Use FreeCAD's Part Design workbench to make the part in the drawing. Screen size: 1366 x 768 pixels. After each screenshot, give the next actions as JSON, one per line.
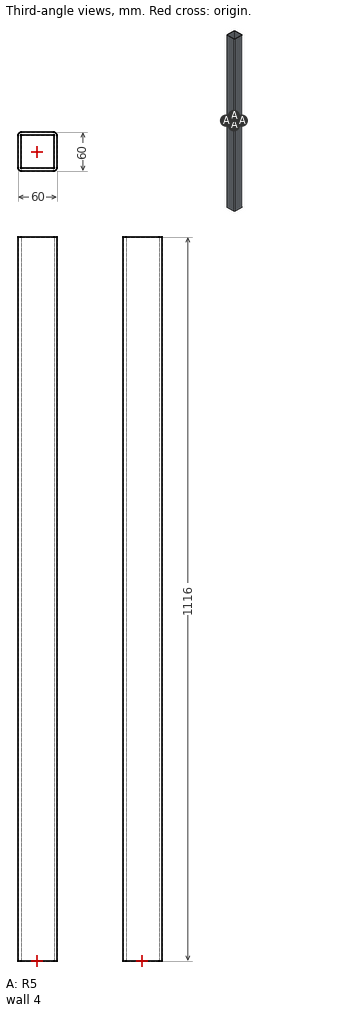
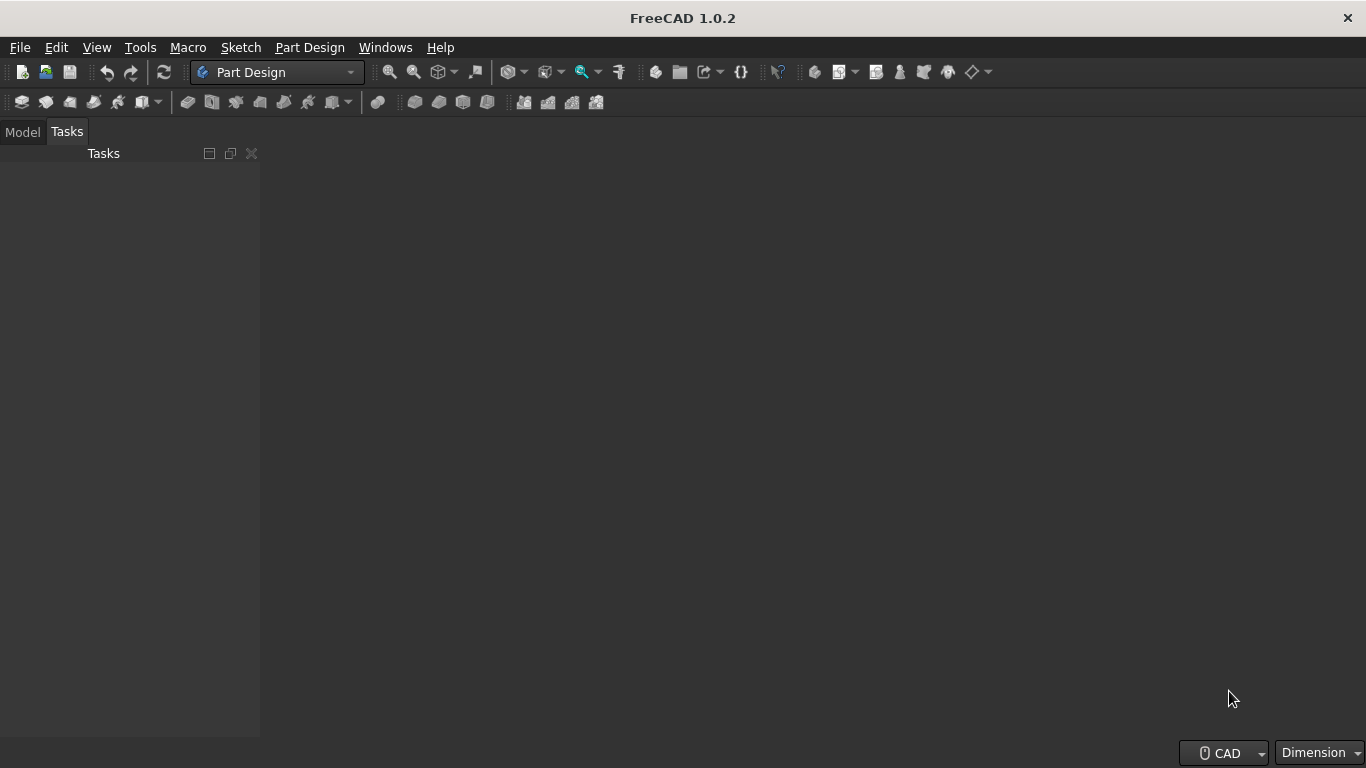
{"action": "left_click", "coordinate": [22, 72]}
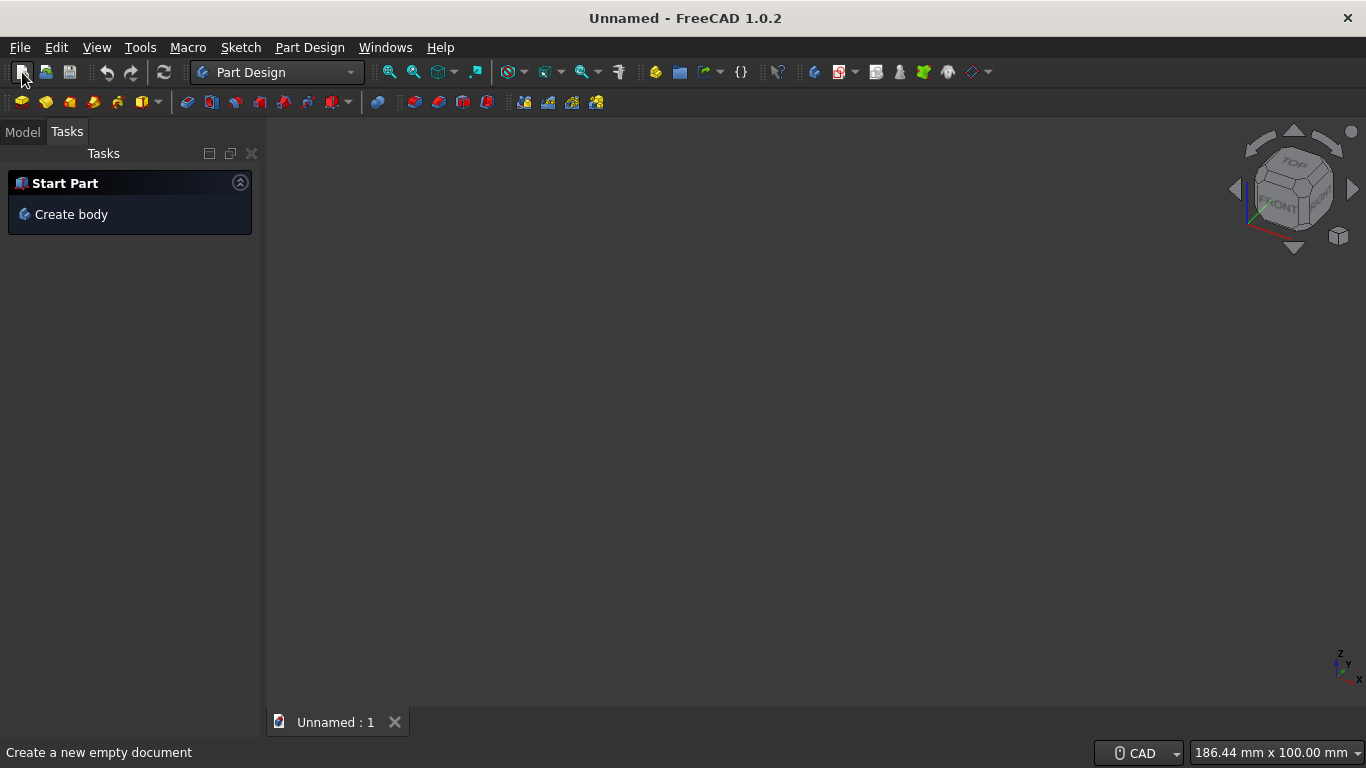
{"action": "left_click", "coordinate": [840, 72]}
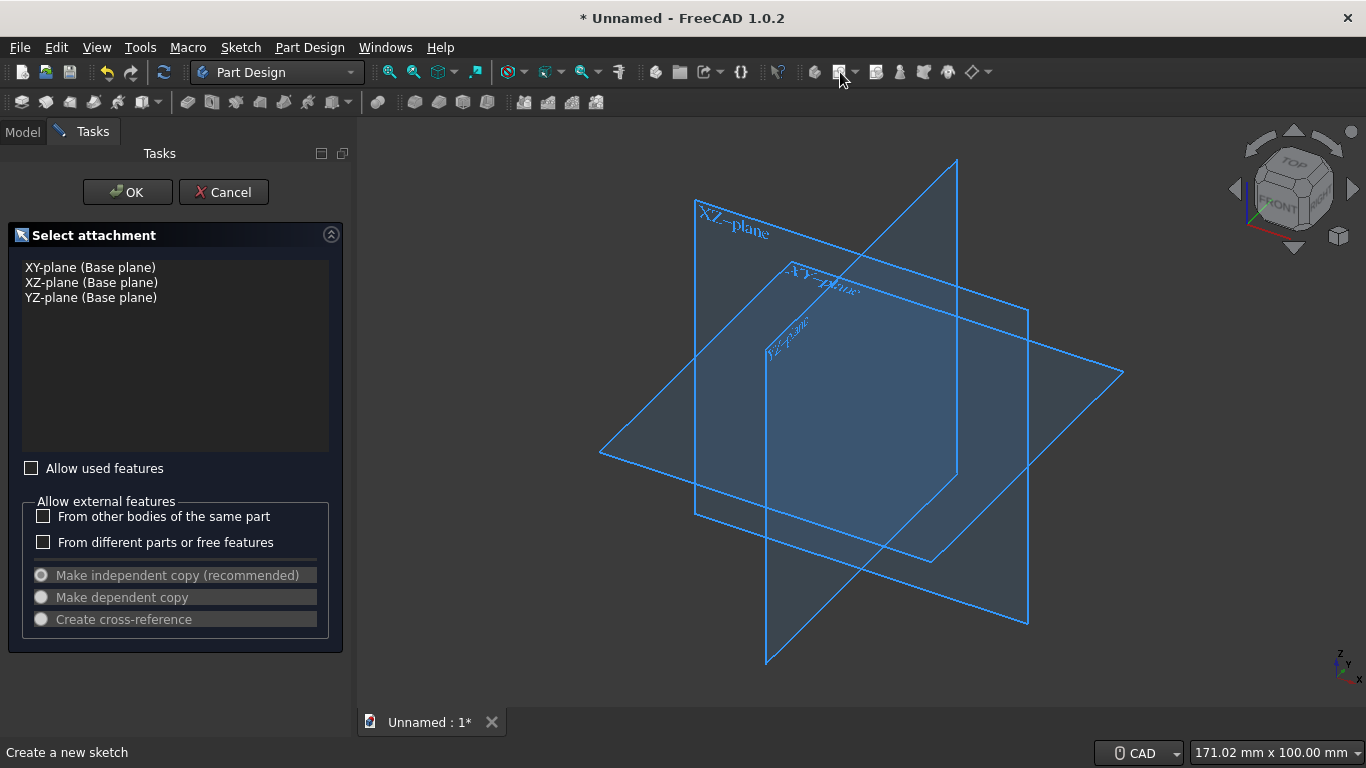
{"action": "left_click", "coordinate": [82, 268]}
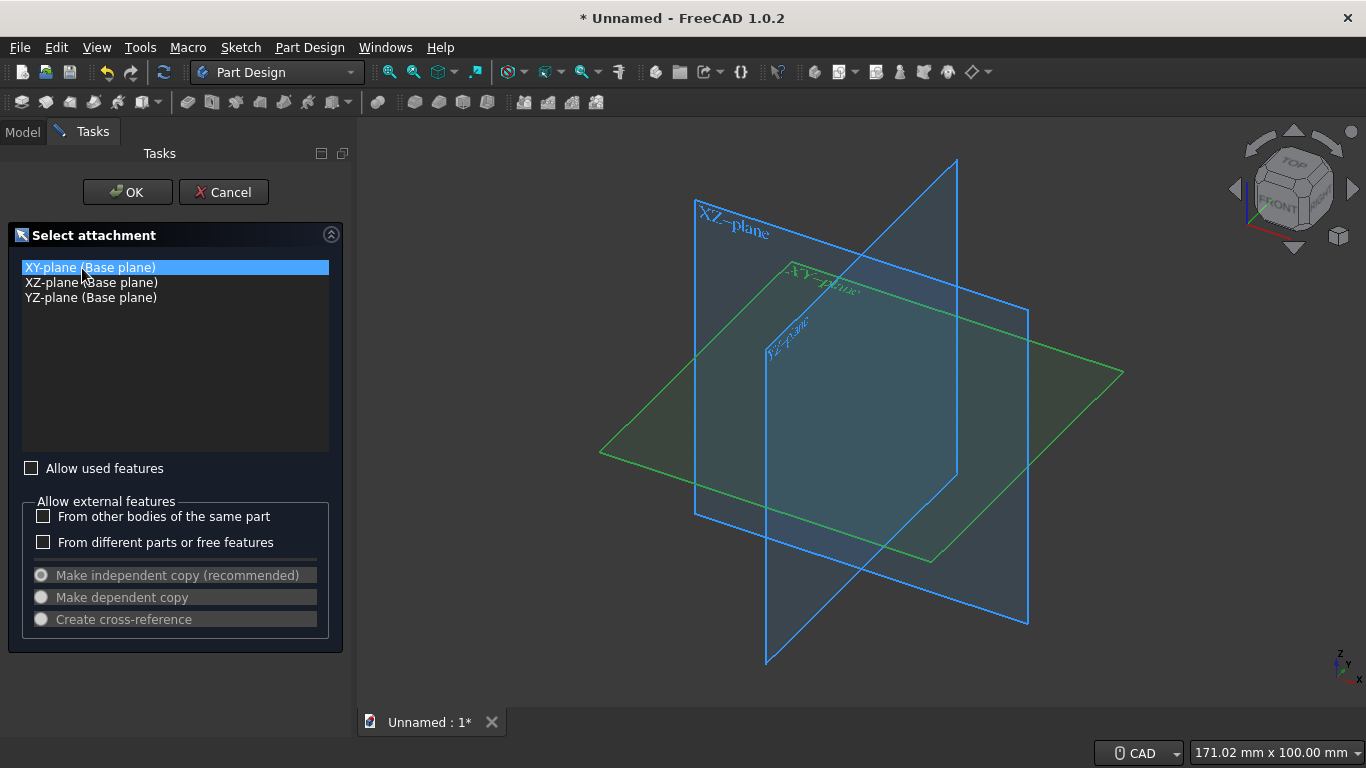
{"action": "left_click", "coordinate": [128, 192]}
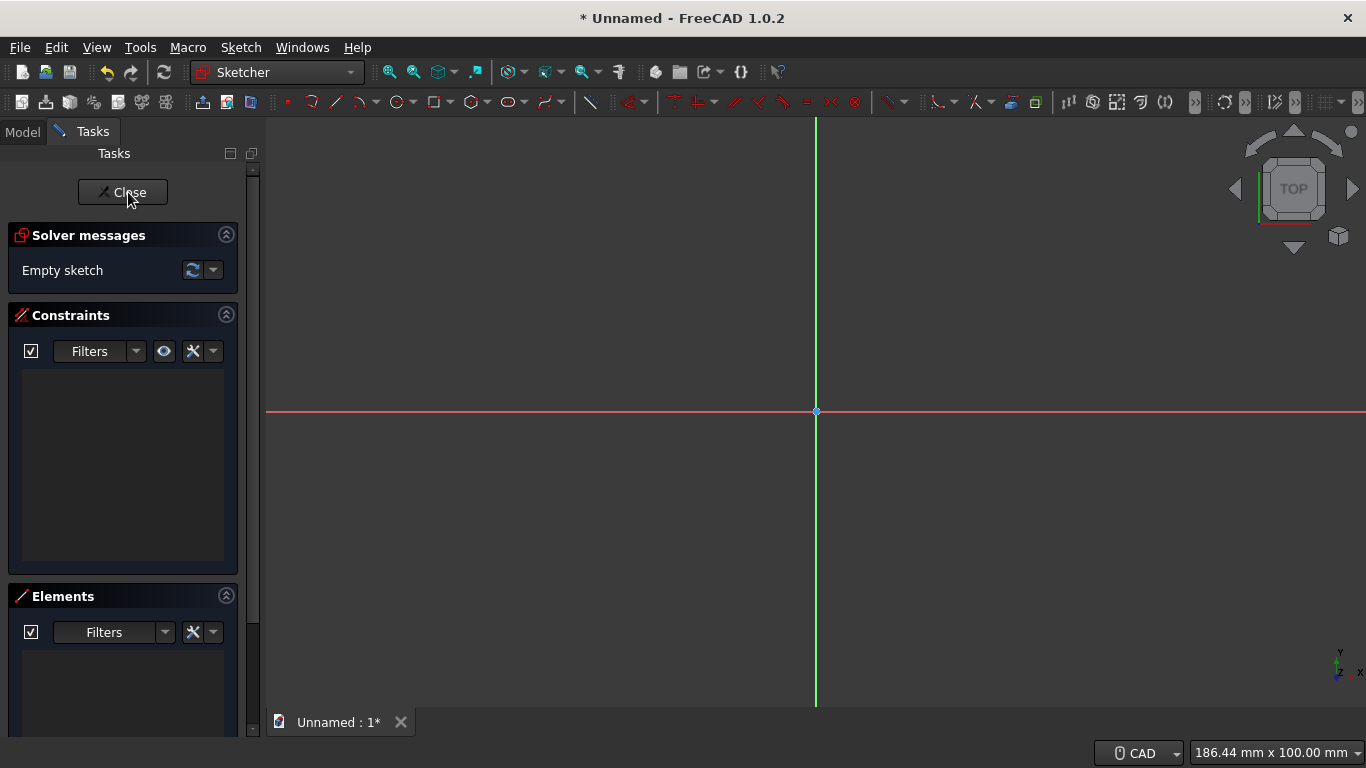
{"action": "left_click", "coordinate": [452, 102]}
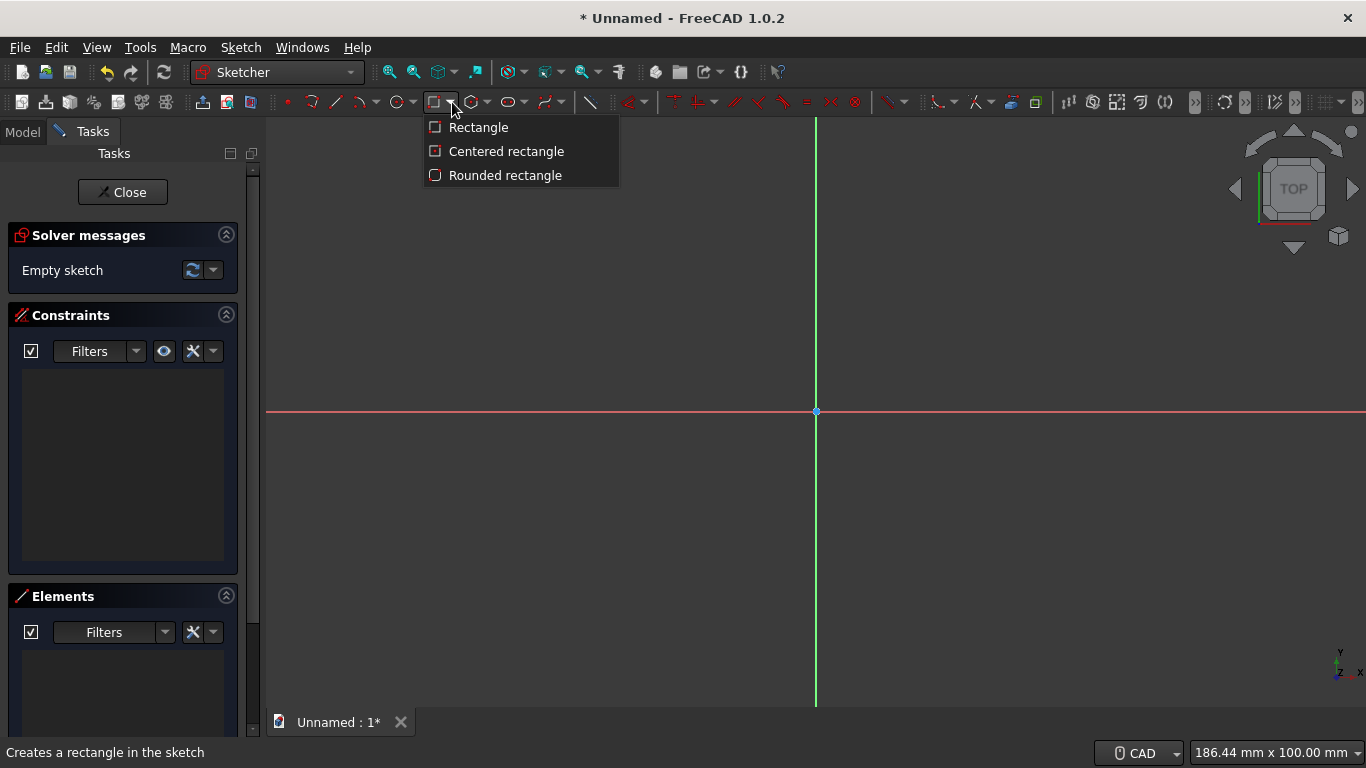
{"action": "left_click", "coordinate": [522, 151]}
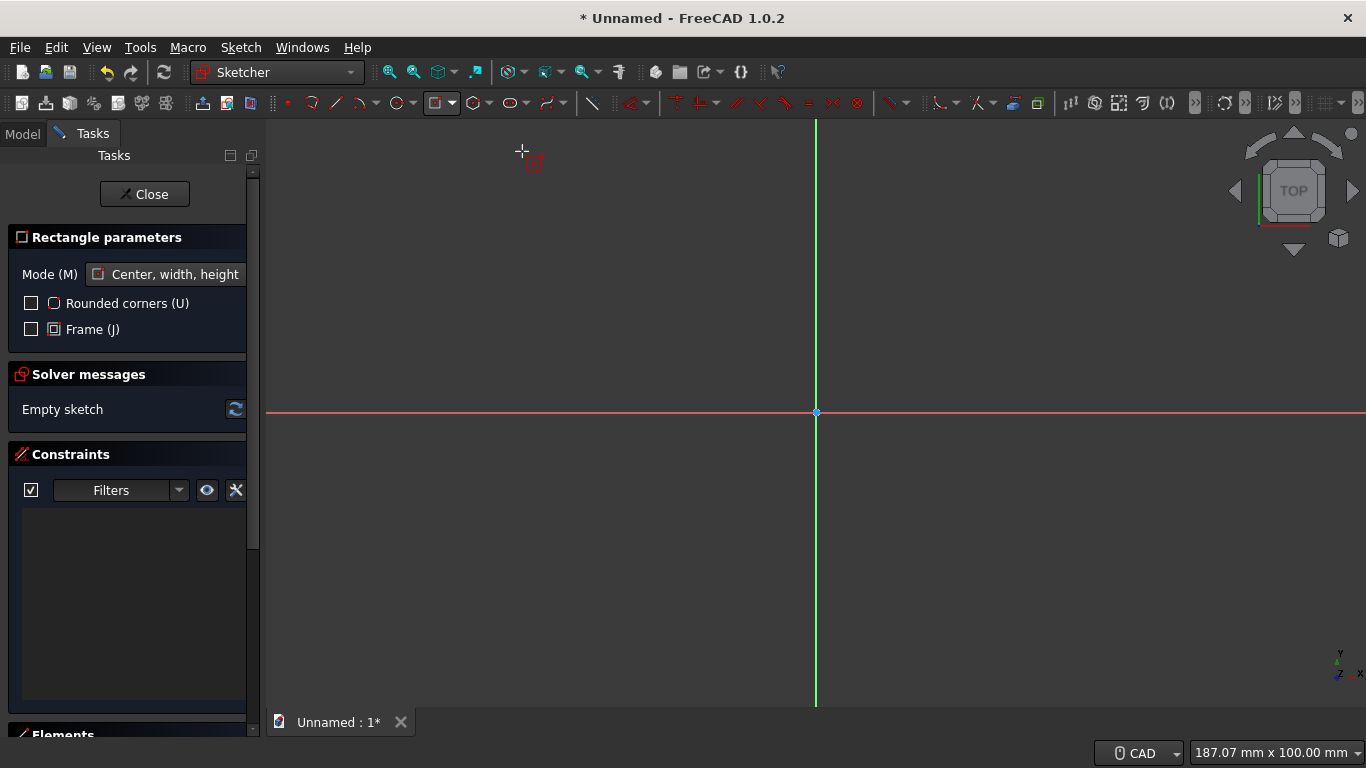
{"action": "left_click", "coordinate": [816, 413]}
{"action": "left_click", "coordinate": [992, 237]}
{"action": "key", "text": "Escape"}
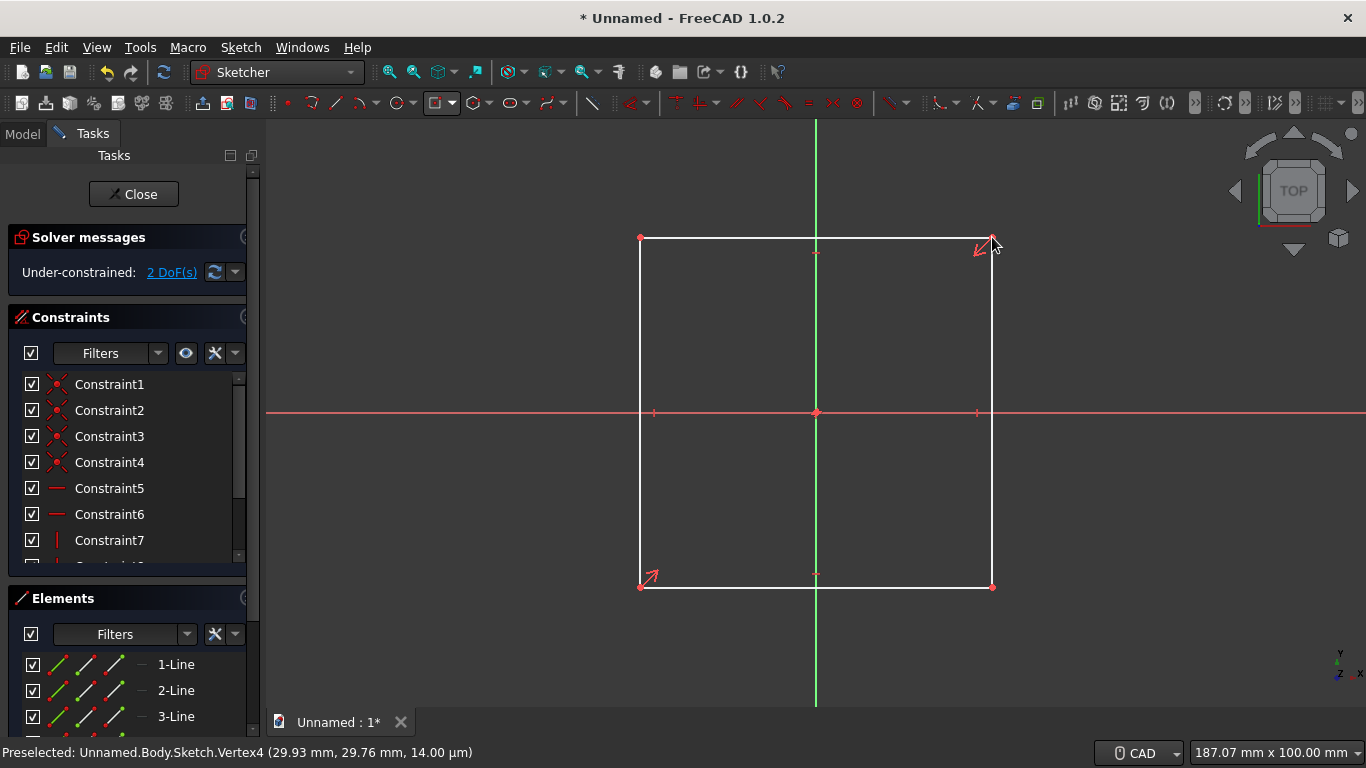
{"action": "left_click", "coordinate": [630, 104]}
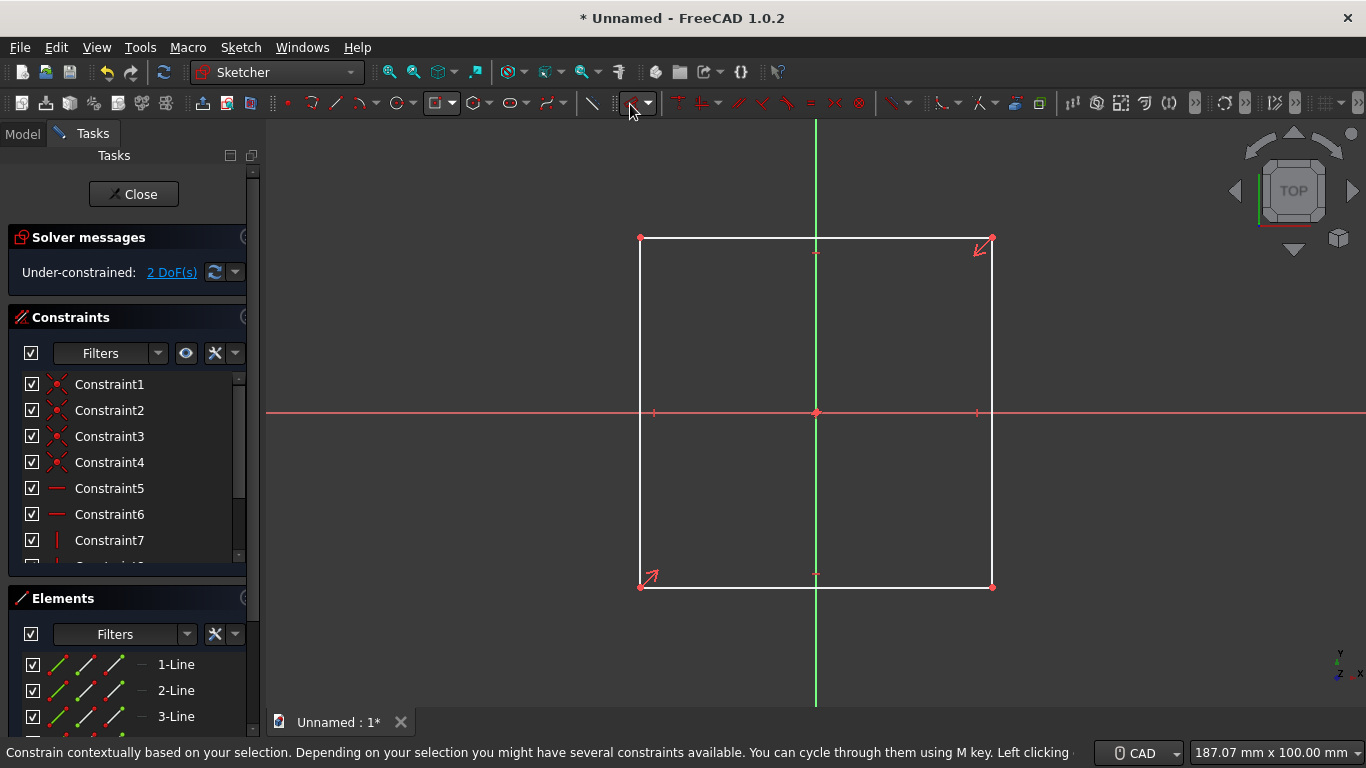
{"action": "left_click", "coordinate": [746, 588]}
{"action": "left_click", "coordinate": [735, 622]}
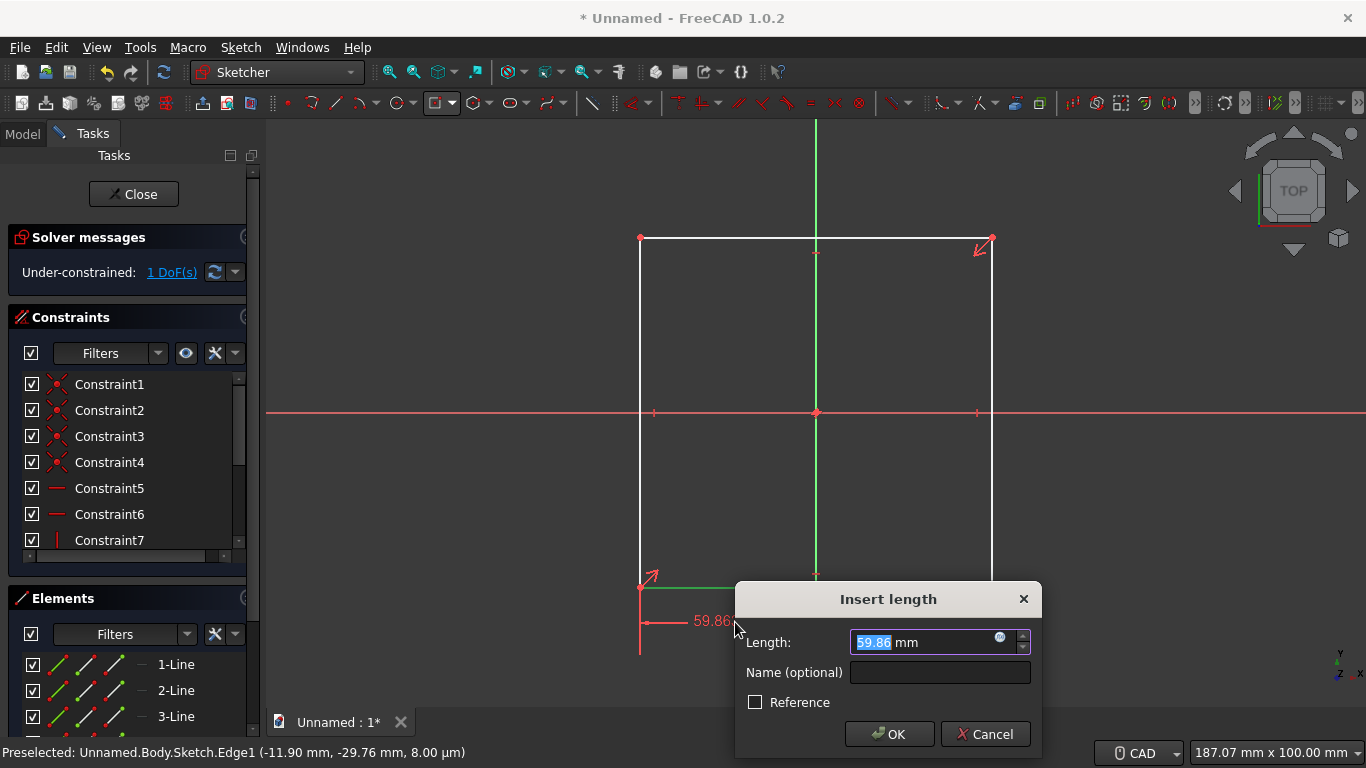
{"action": "type", "text": "60"}
{"action": "key", "text": "Return"}